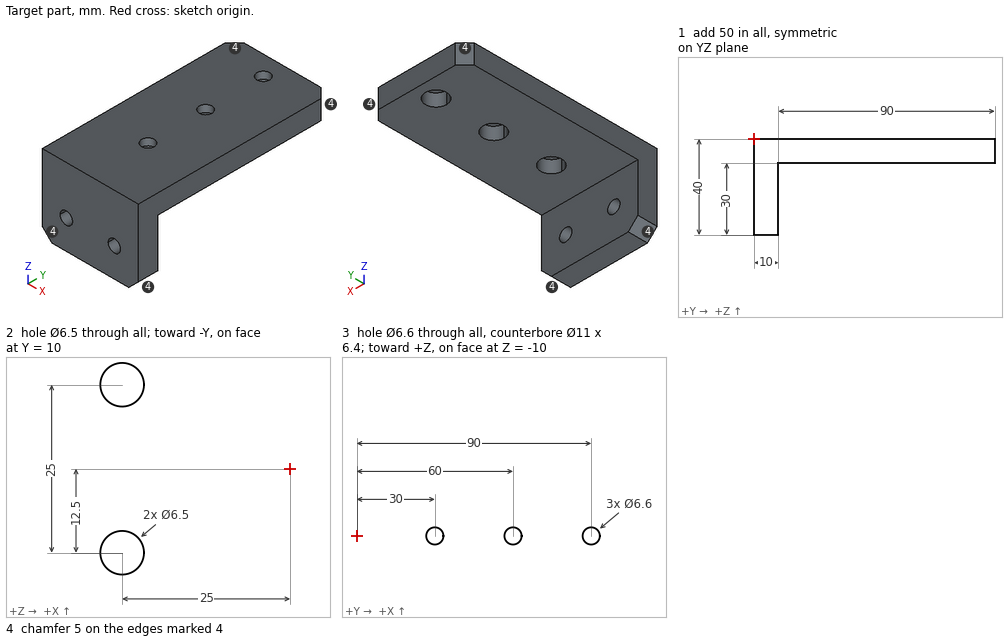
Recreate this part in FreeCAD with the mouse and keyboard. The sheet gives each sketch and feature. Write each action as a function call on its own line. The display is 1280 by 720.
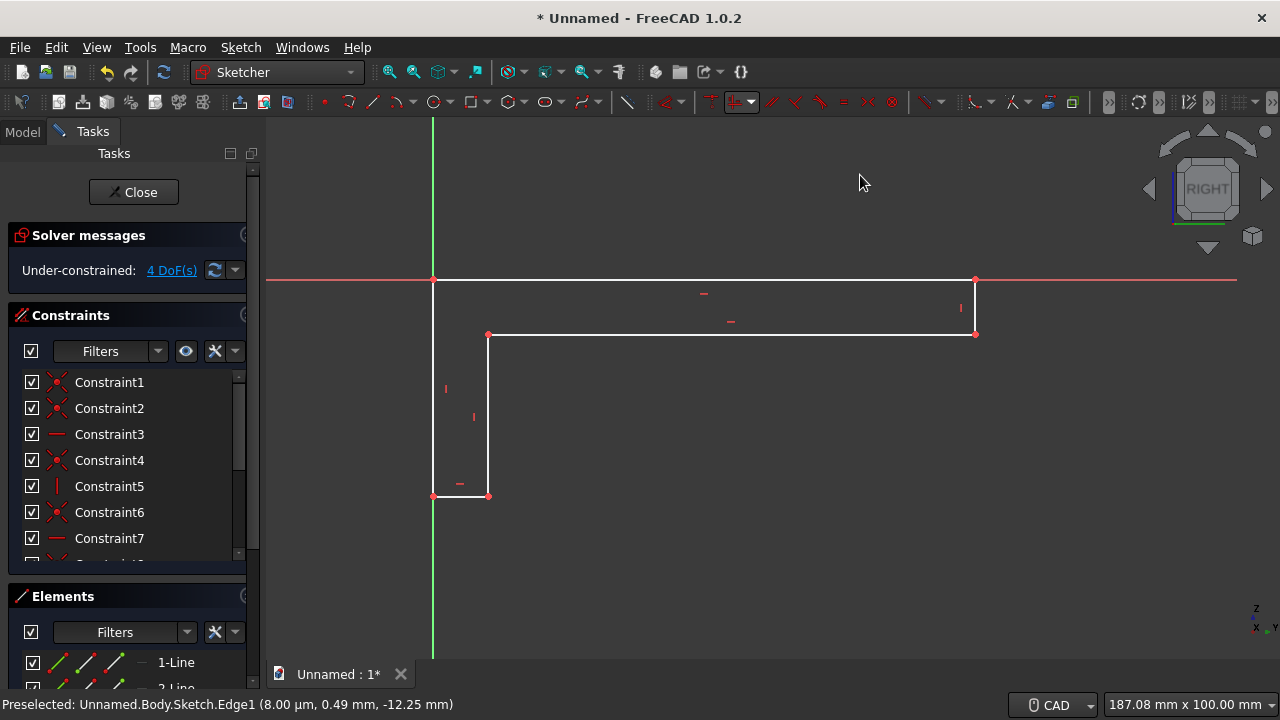
click(433, 345)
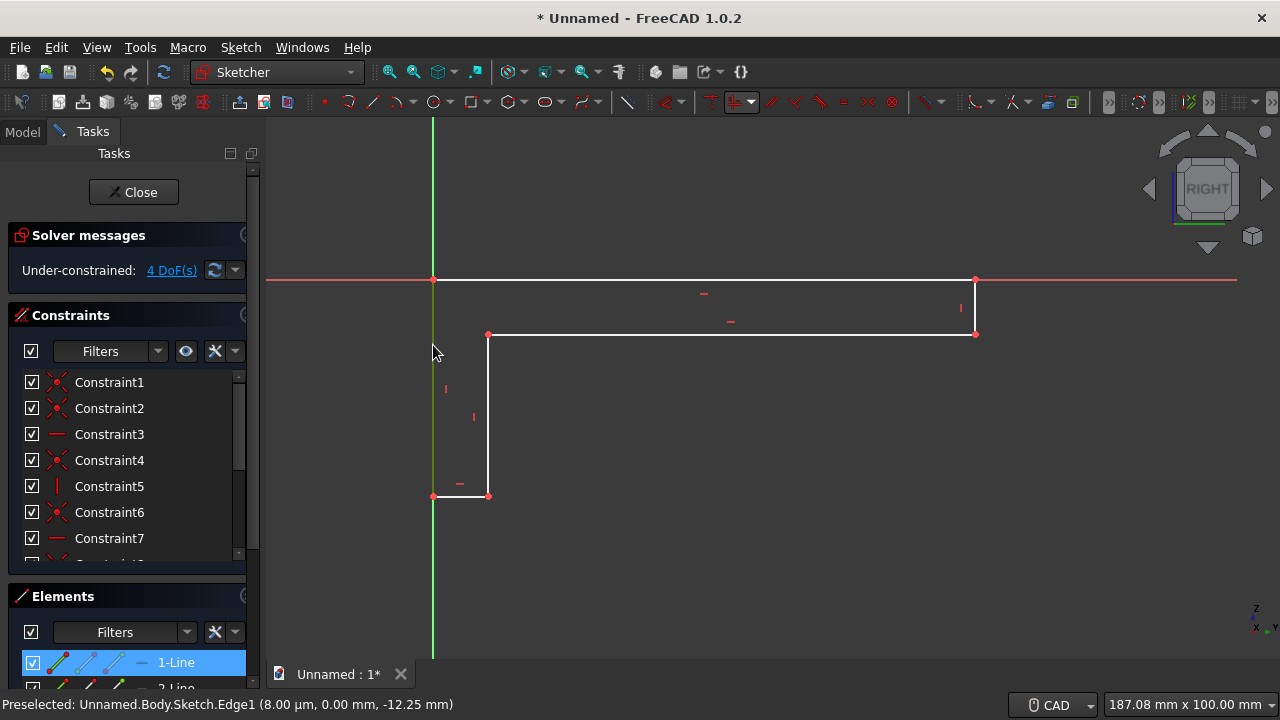
key(i)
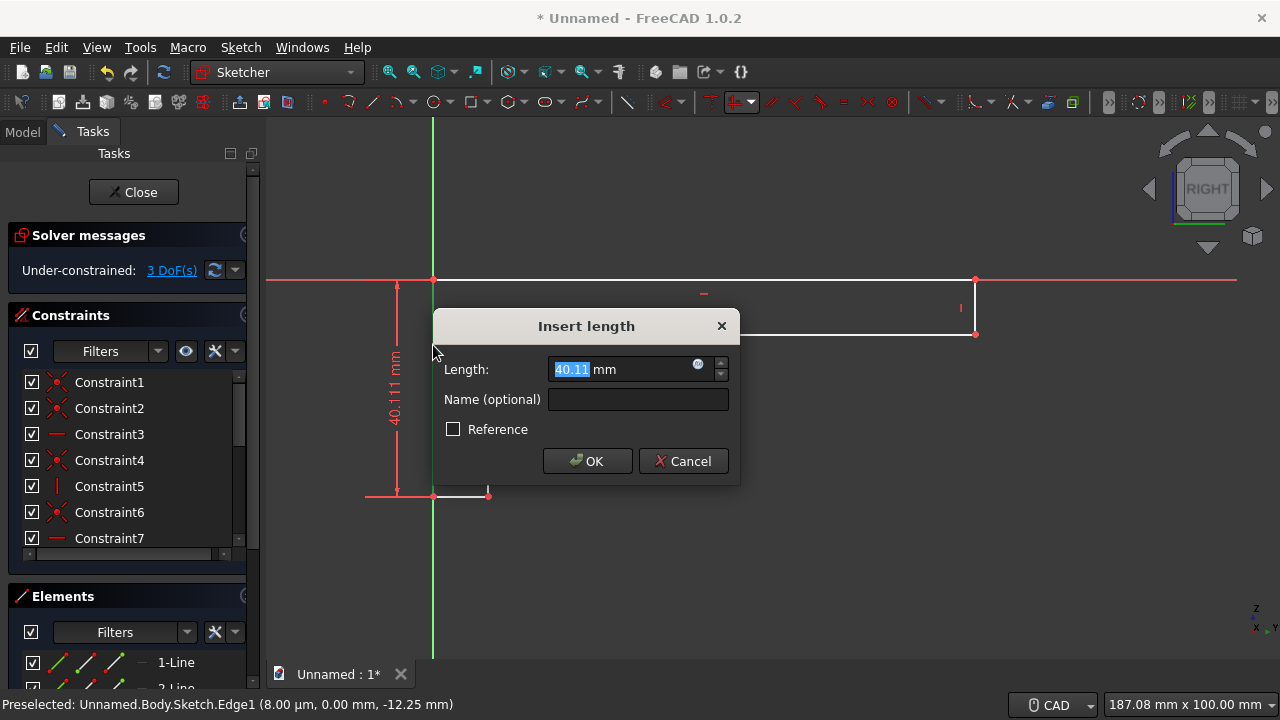
text(40)
key(Return)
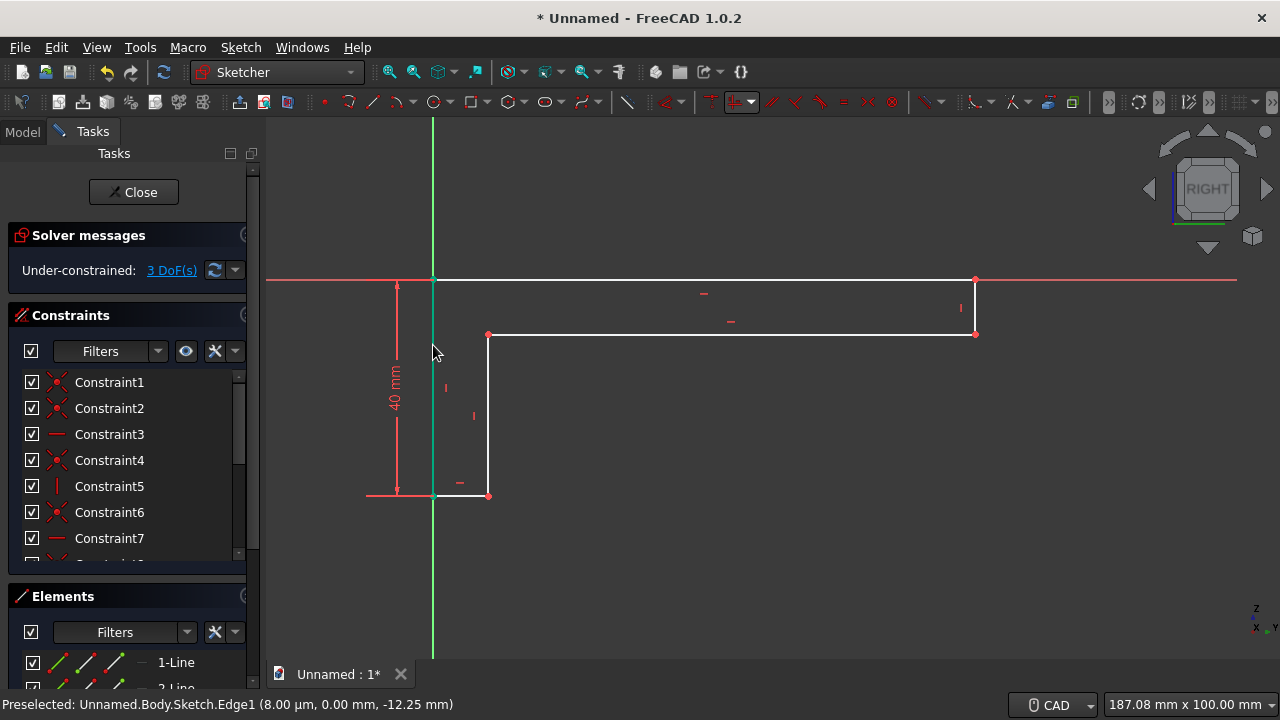
click(450, 496)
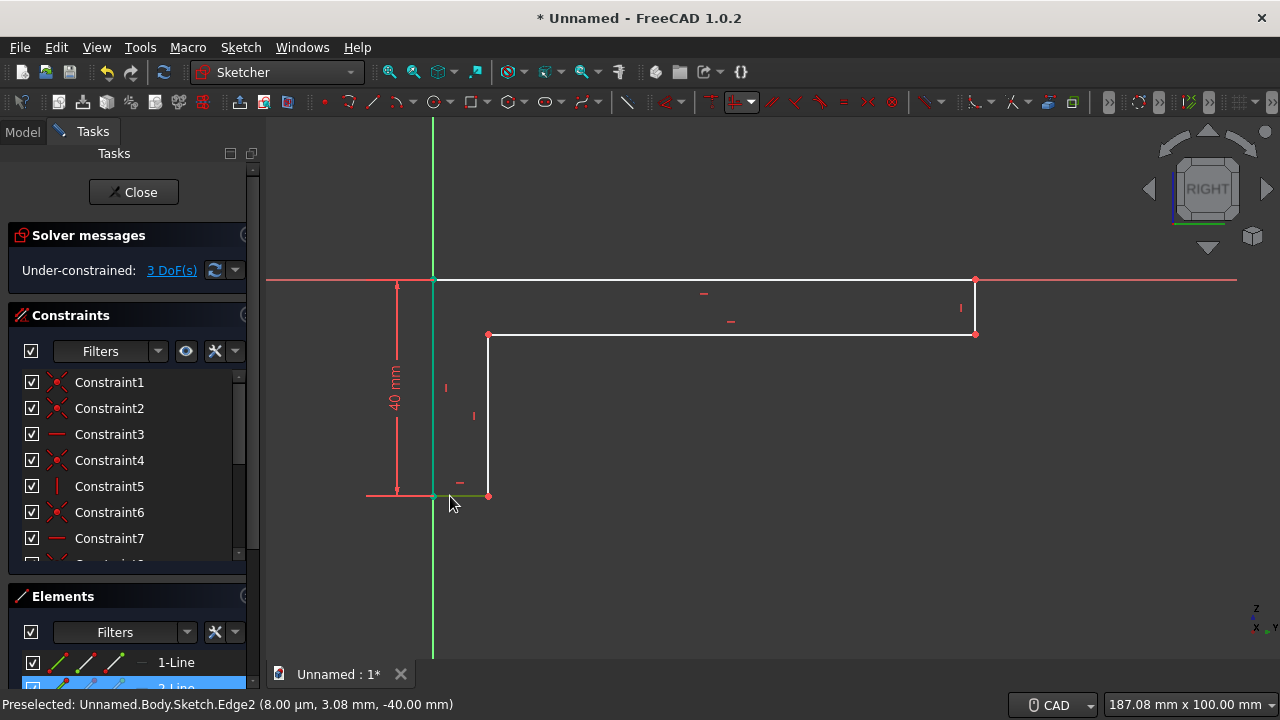
click(684, 102)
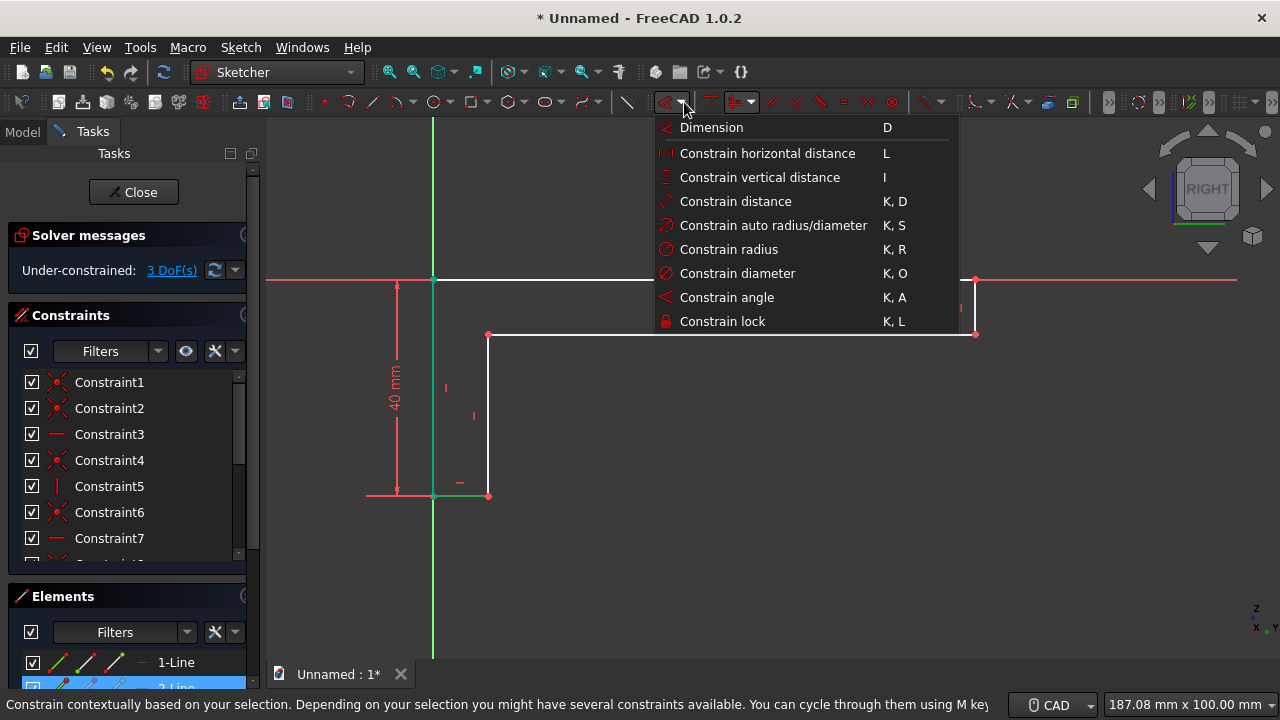
click(807, 153)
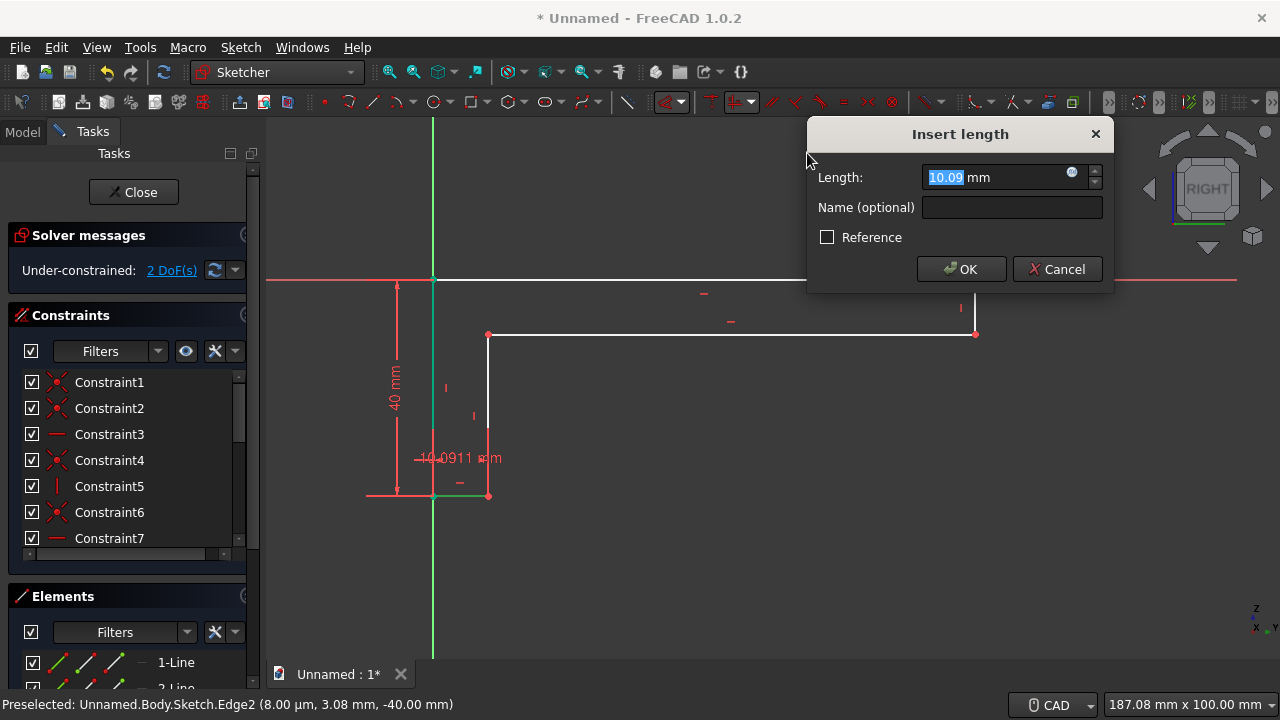
text(10)
key(Return)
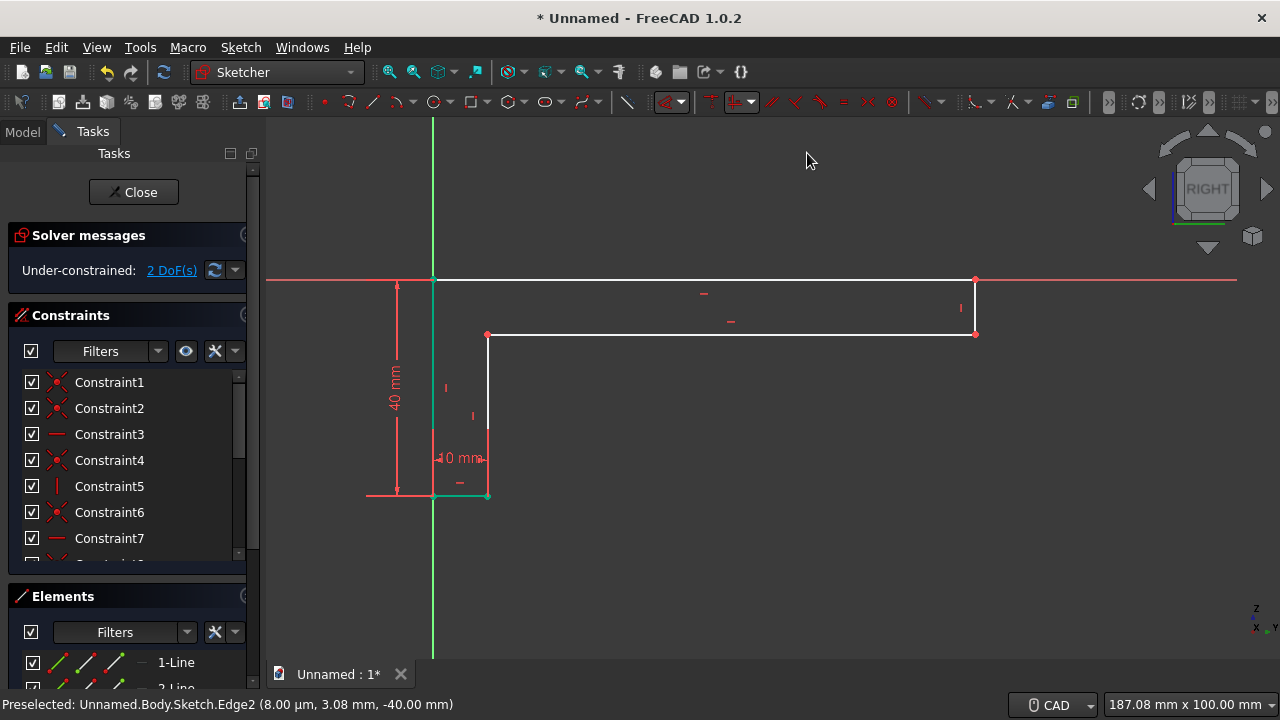
click(488, 448)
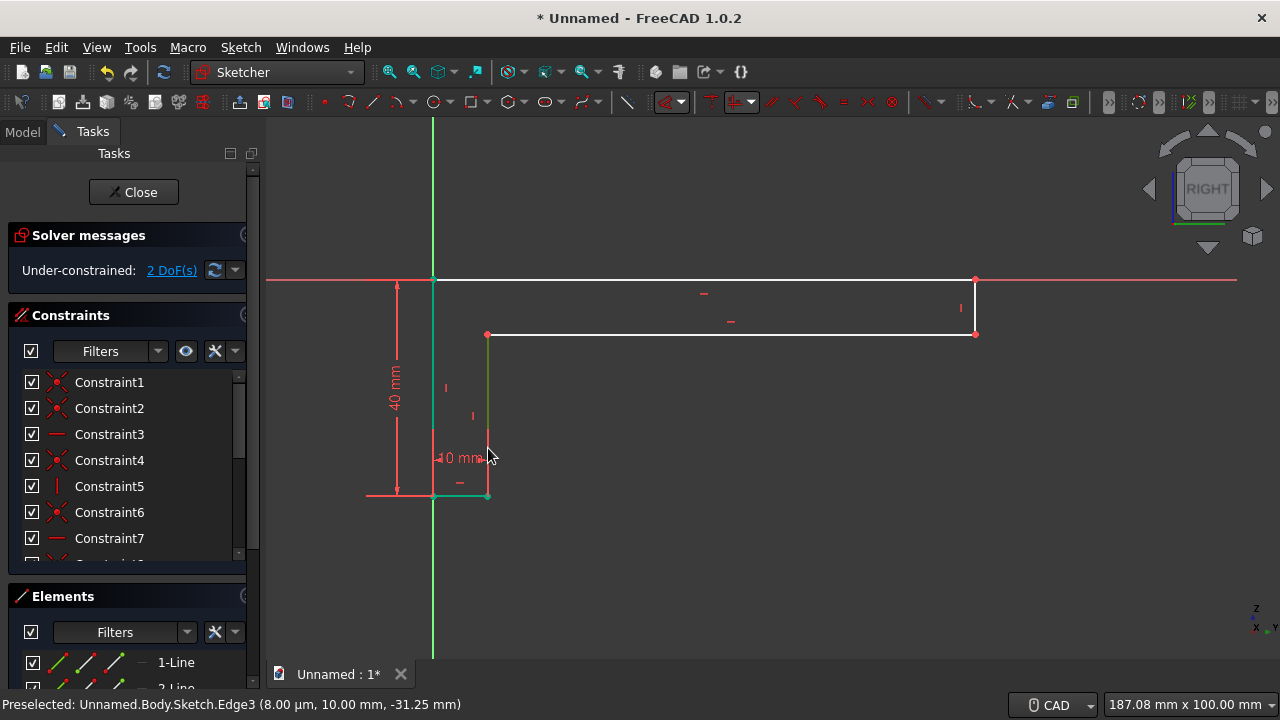
click(684, 102)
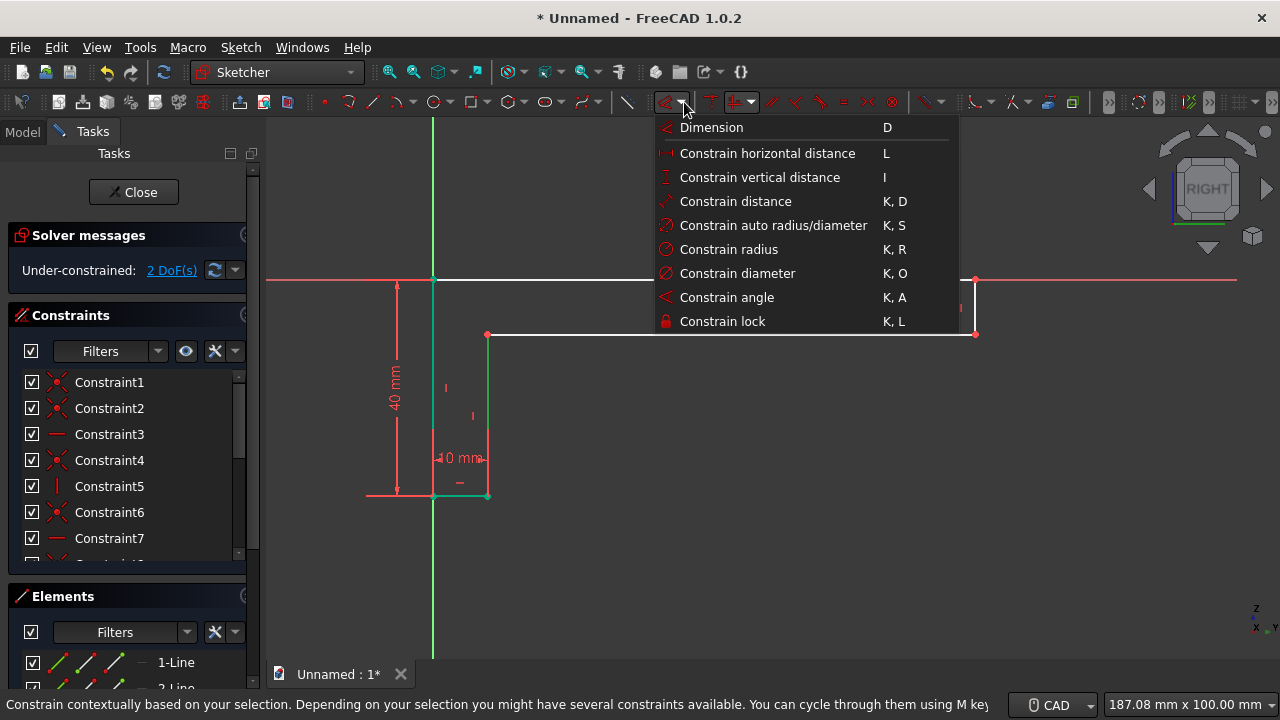
click(807, 177)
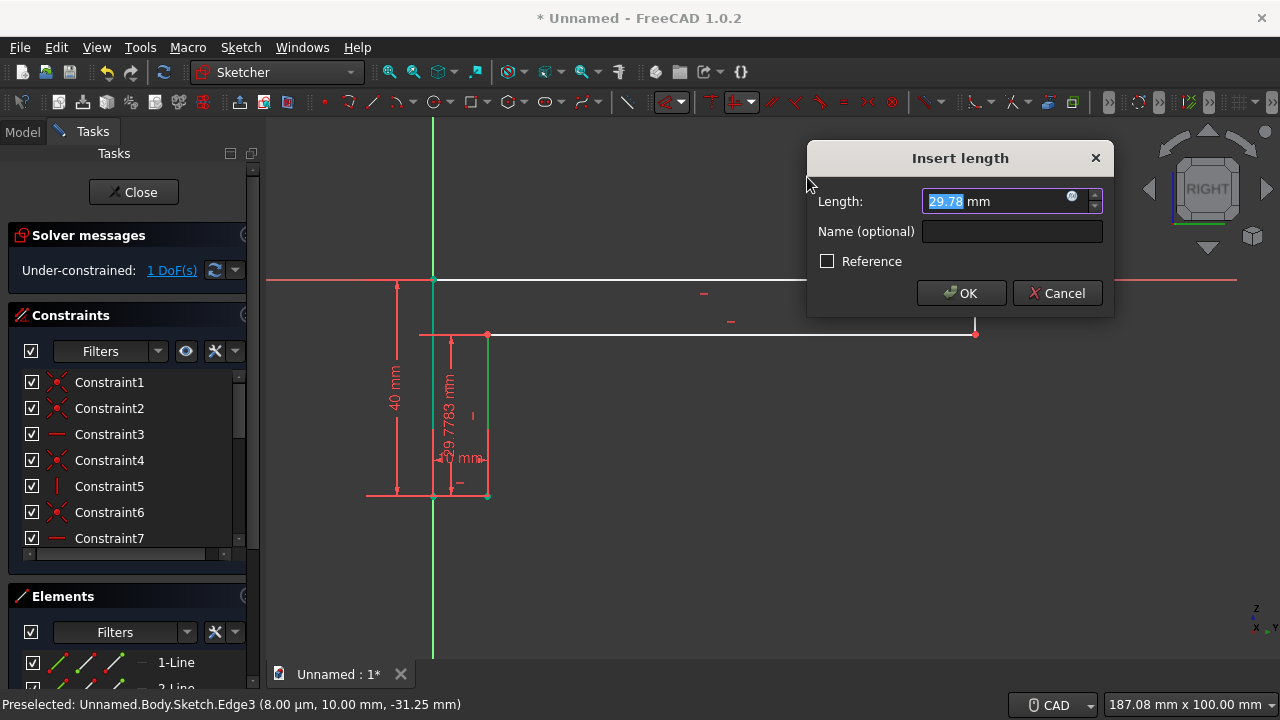
text(30)
key(Return)